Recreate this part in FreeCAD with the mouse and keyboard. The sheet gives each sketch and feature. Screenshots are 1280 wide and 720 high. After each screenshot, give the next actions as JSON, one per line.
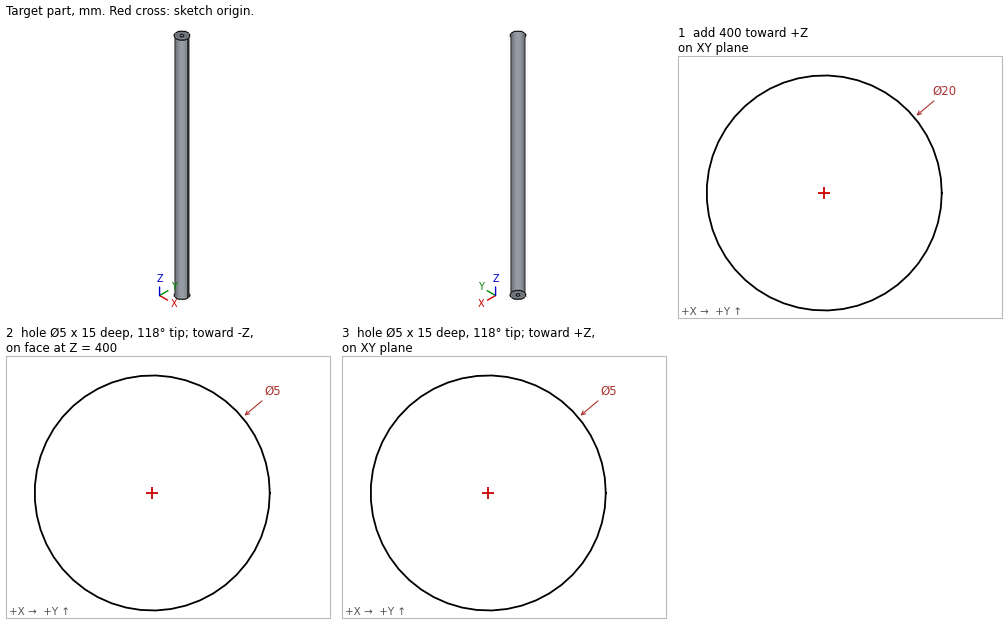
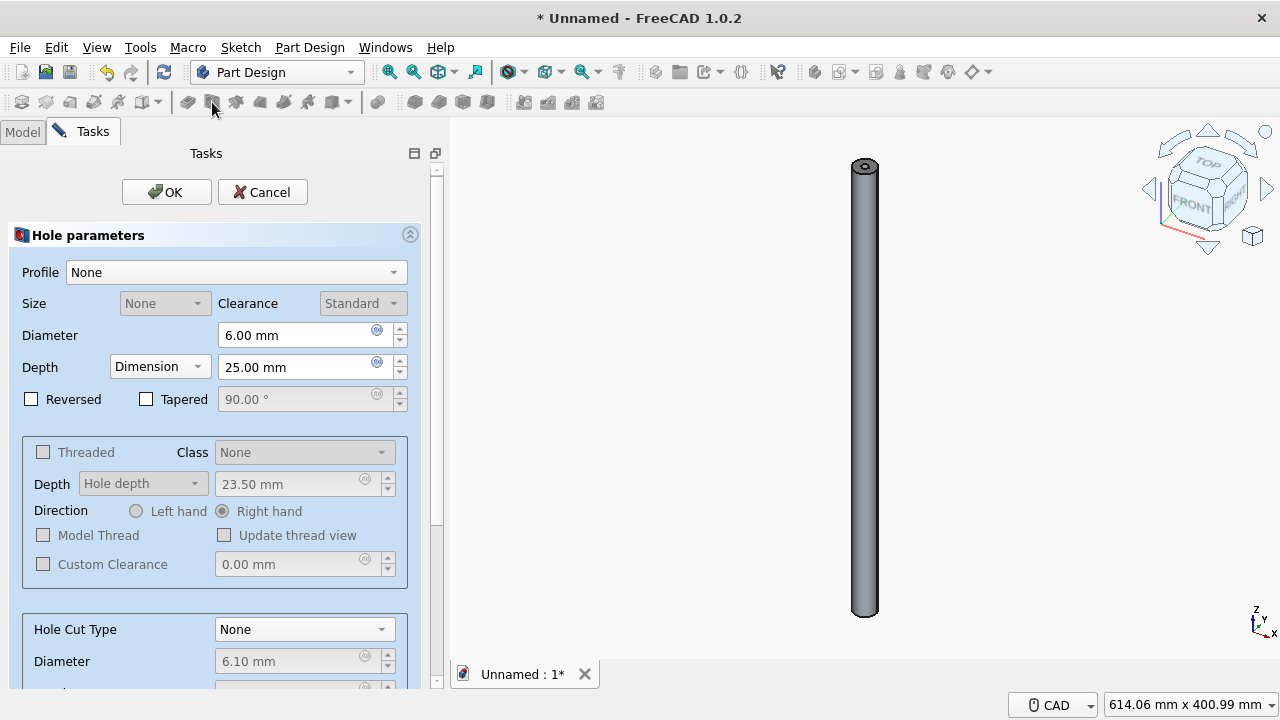
{"action": "triple_click", "coordinate": [305, 335]}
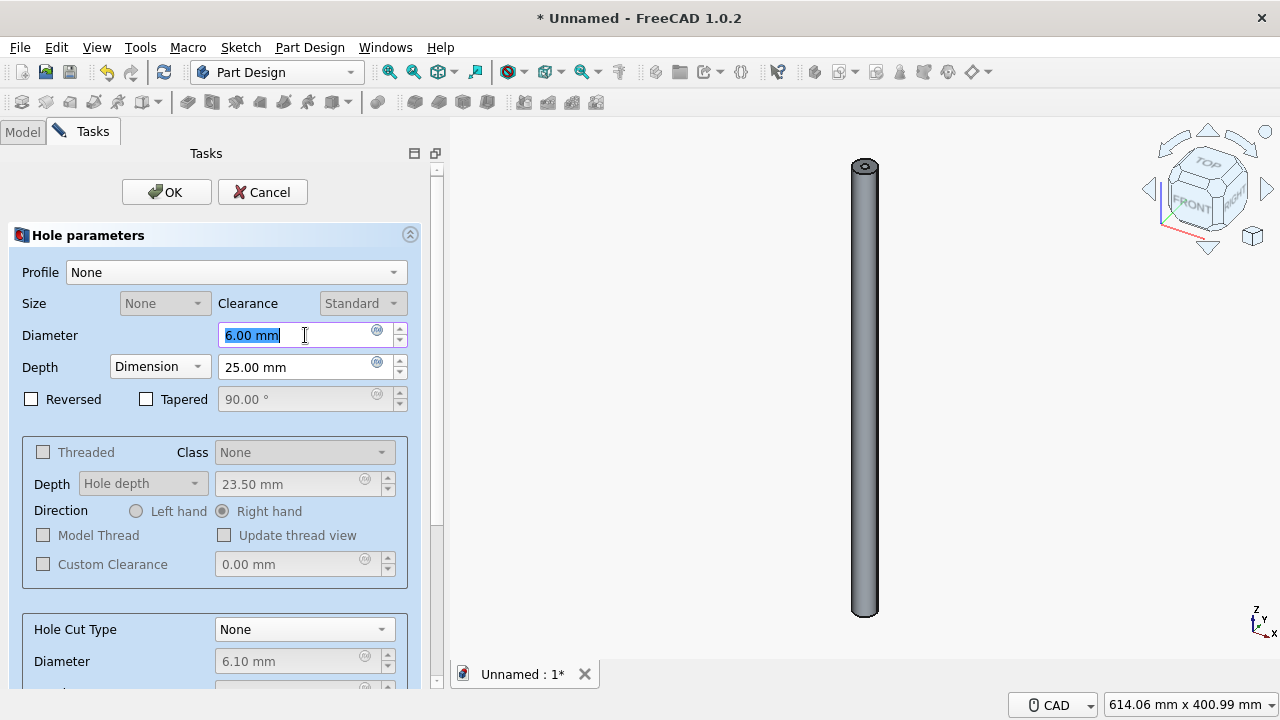
{"action": "type", "text": "5"}
{"action": "key", "text": "Tab"}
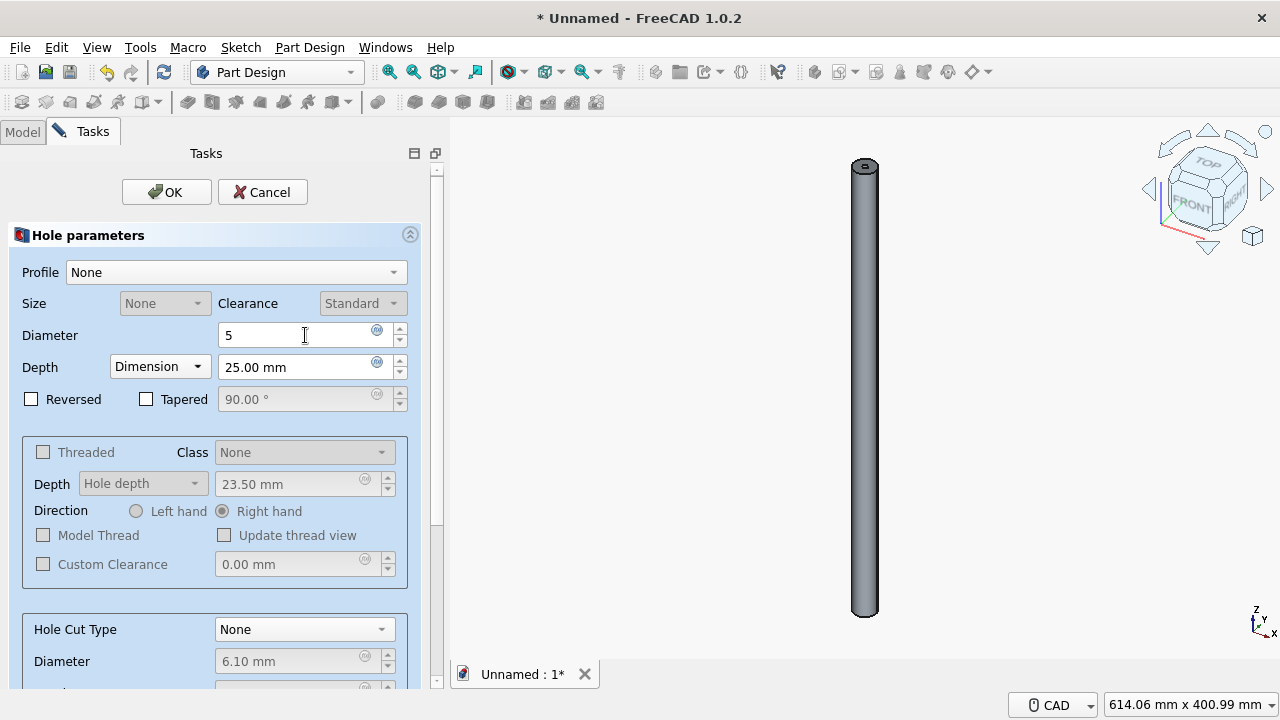
{"action": "triple_click", "coordinate": [305, 367]}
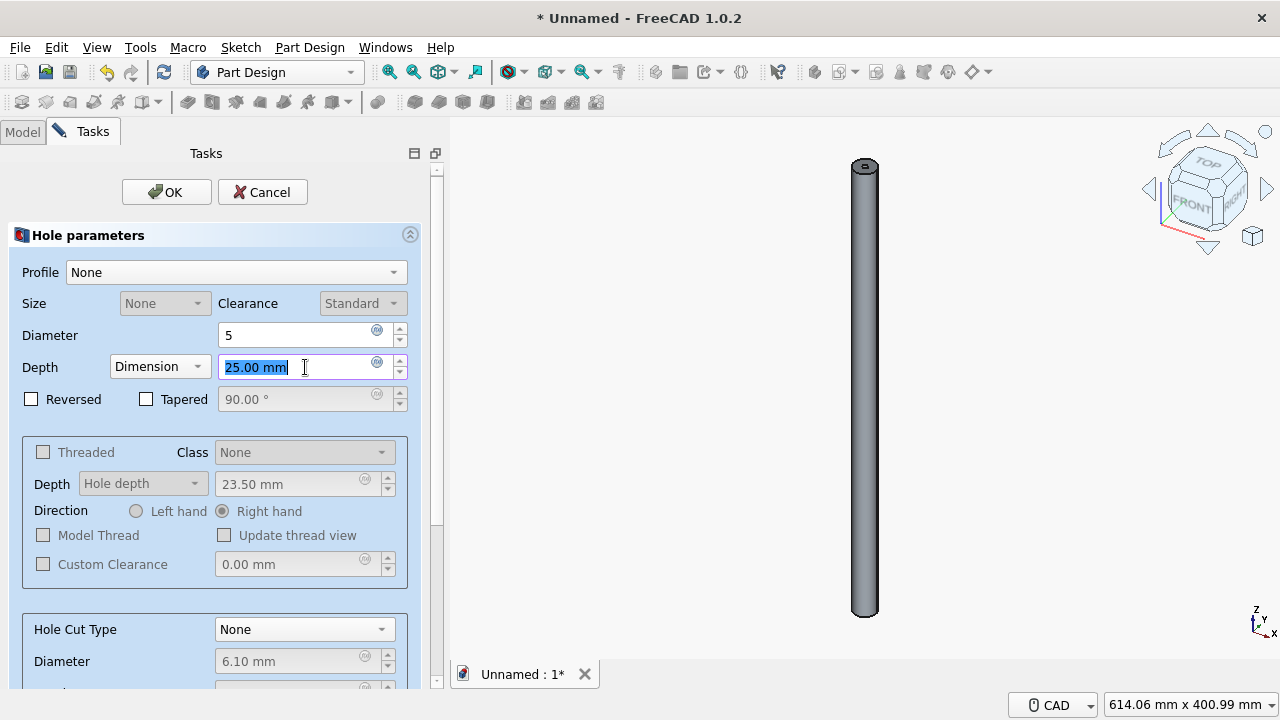
{"action": "type", "text": "15"}
{"action": "key", "text": "Tab"}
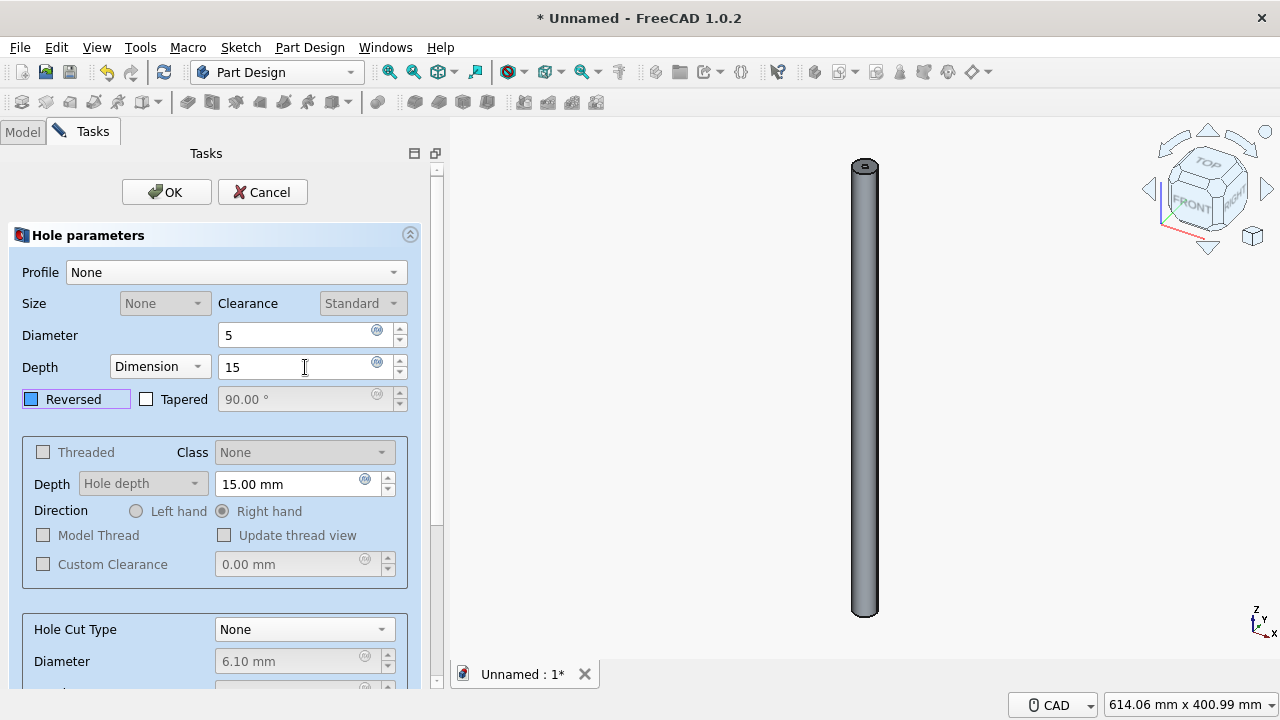
{"action": "left_click", "coordinate": [167, 192]}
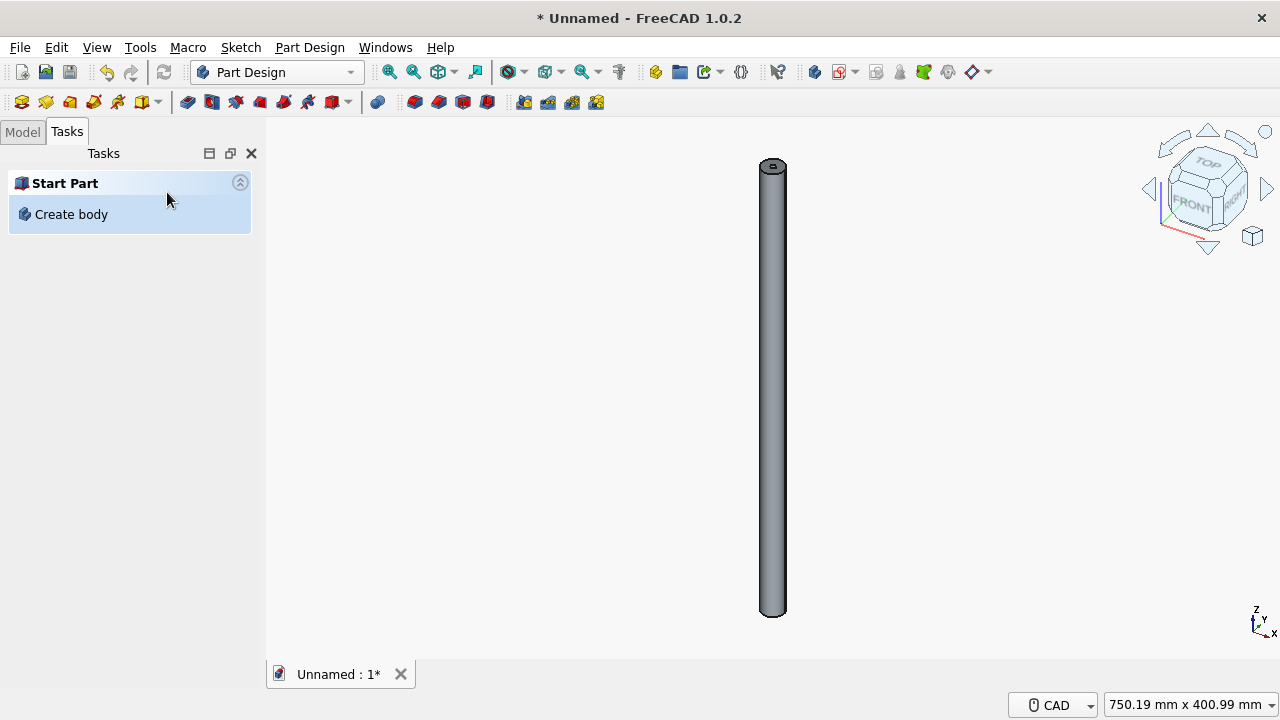
{"action": "left_click", "coordinate": [840, 72]}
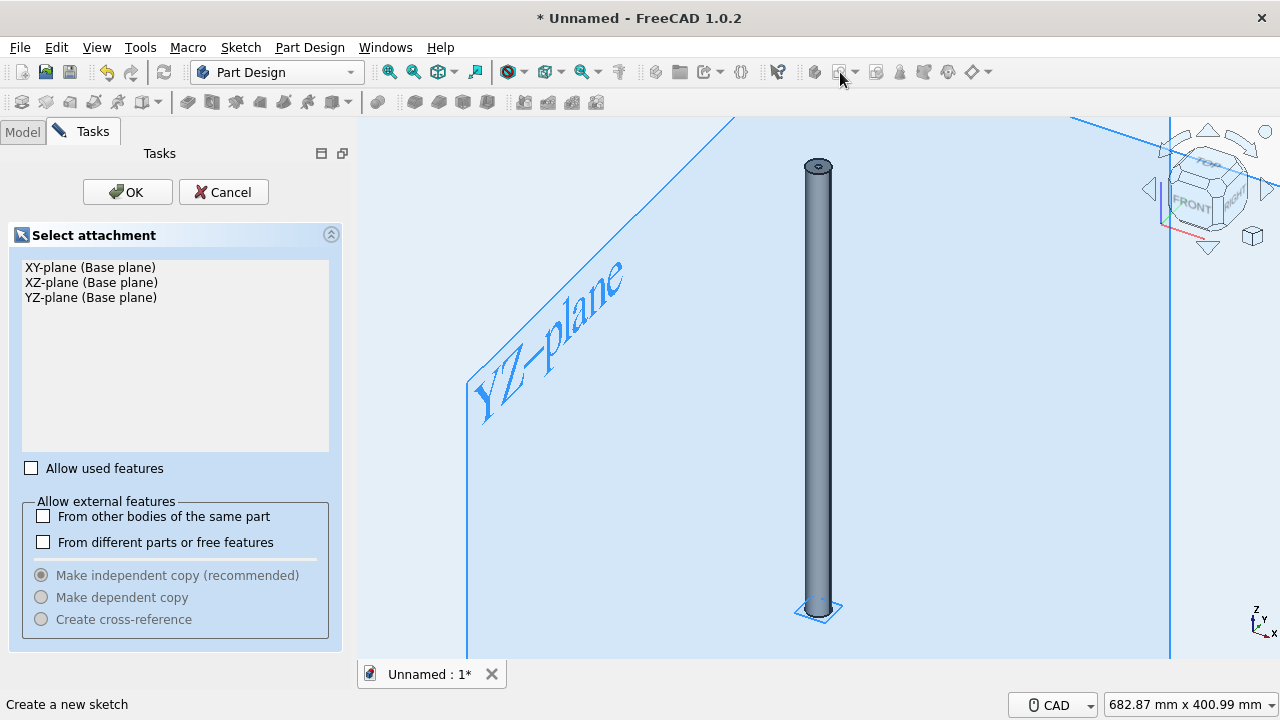
{"action": "left_click", "coordinate": [82, 268]}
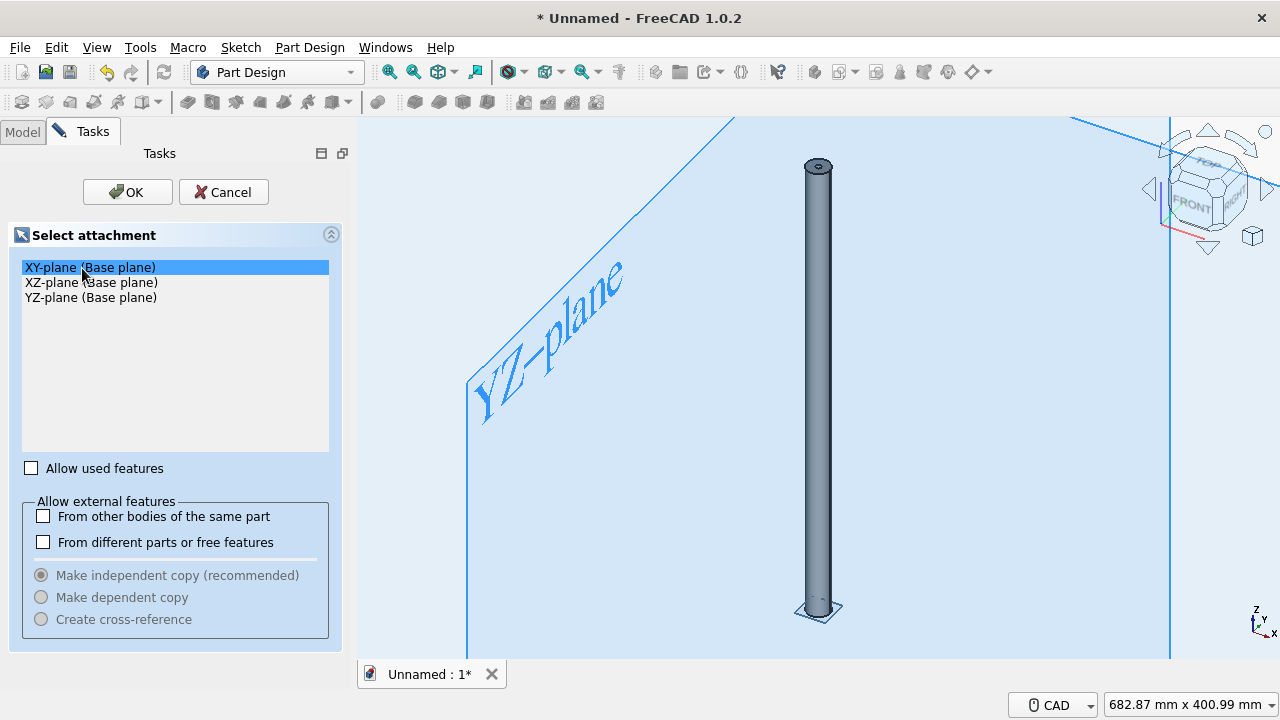
{"action": "left_click", "coordinate": [128, 192]}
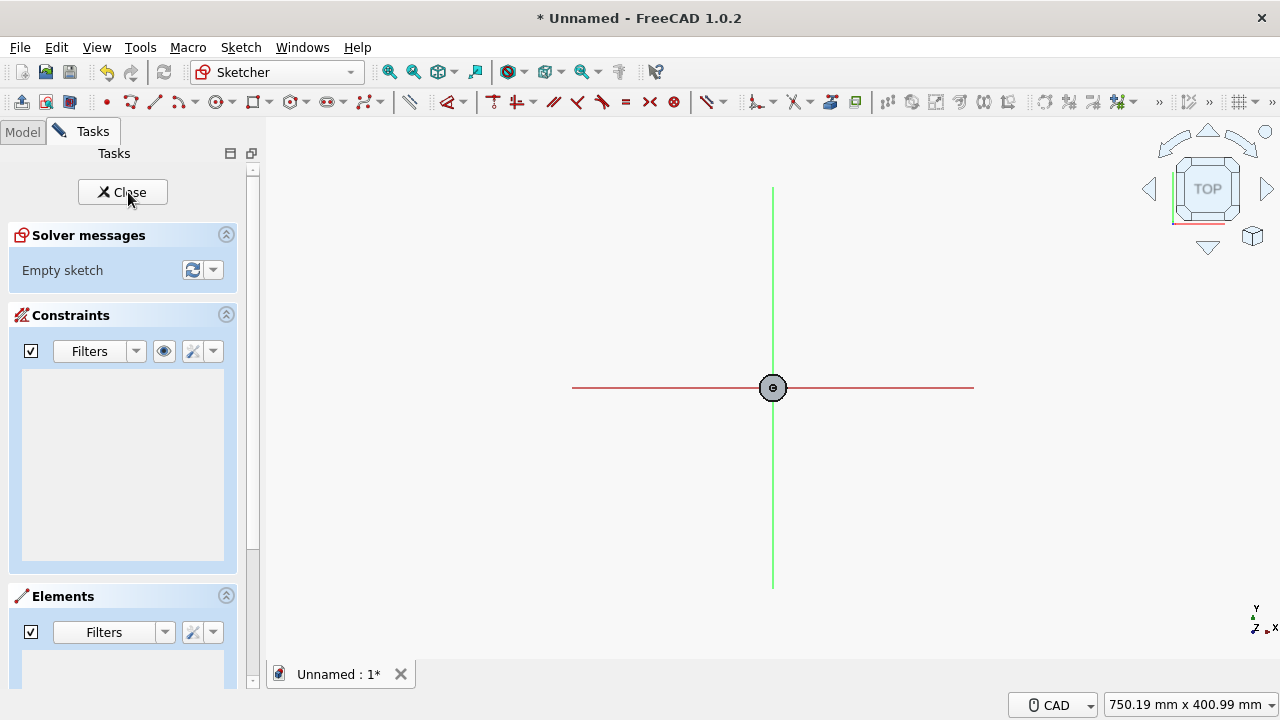
{"action": "left_click", "coordinate": [70, 102]}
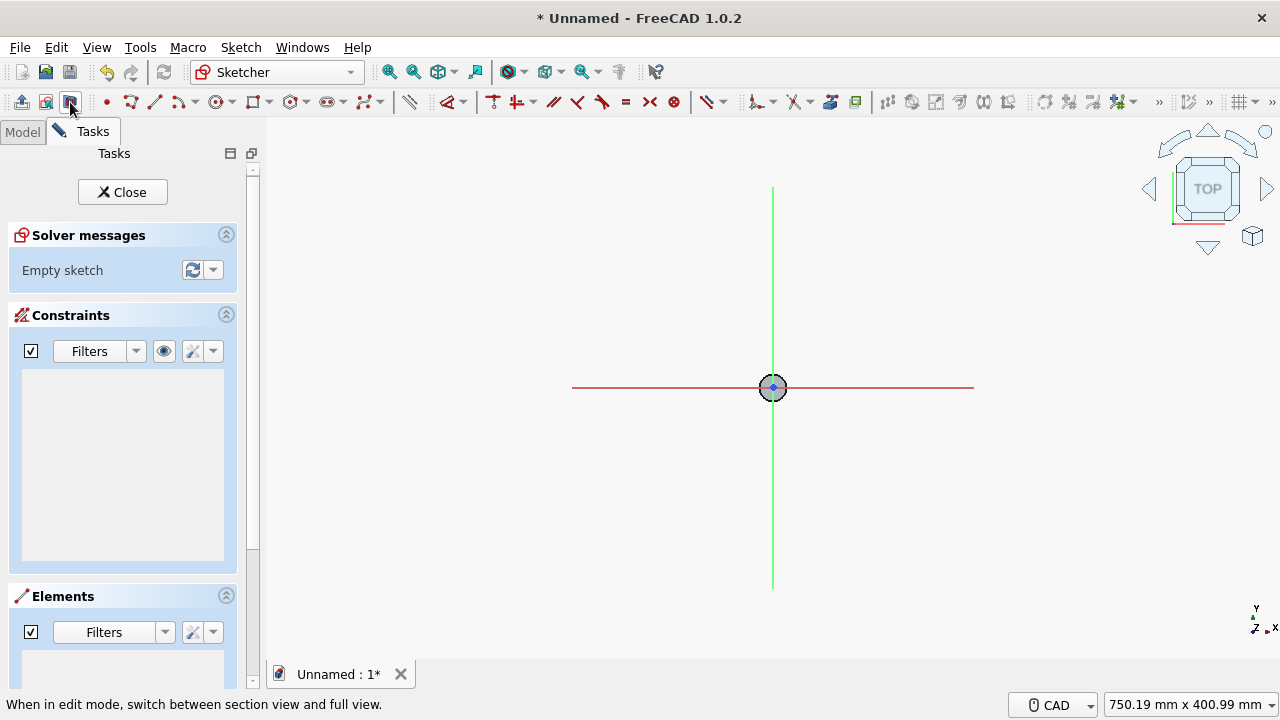
{"action": "scroll", "coordinate": [777, 388], "scroll_direction": "up", "scroll_amount": 15}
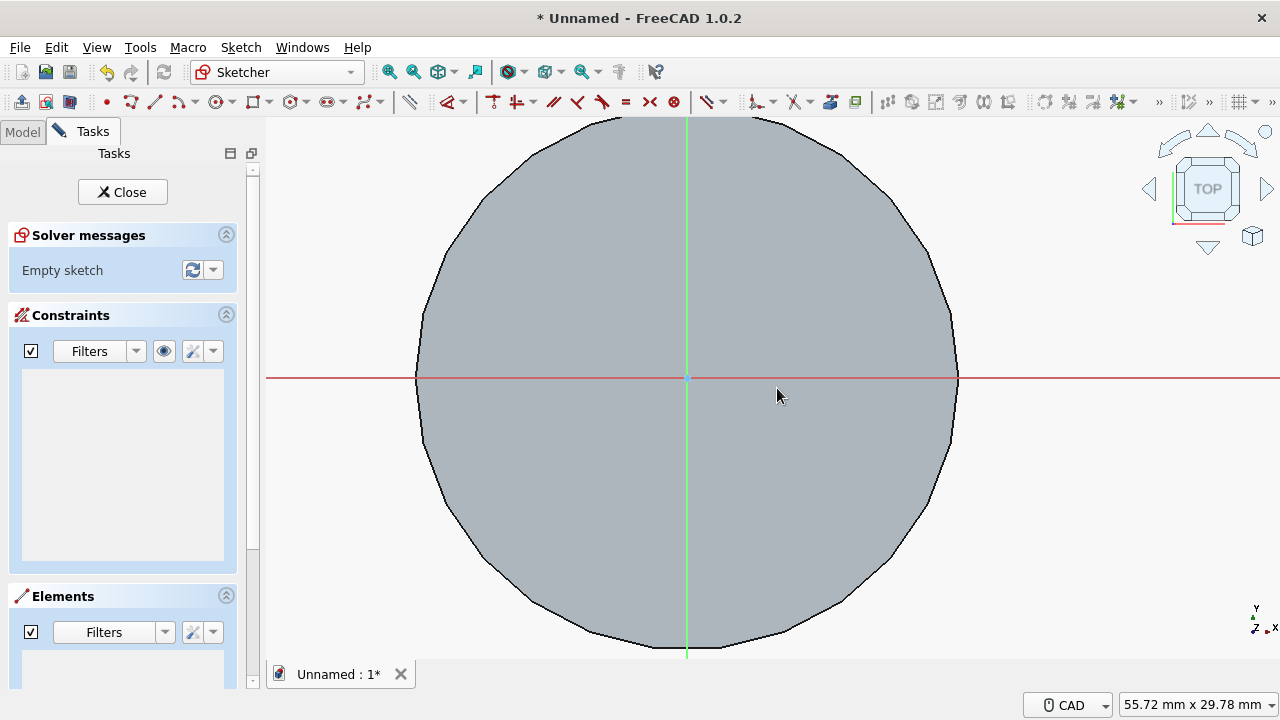
{"action": "scroll", "coordinate": [677, 373], "scroll_direction": "up", "scroll_amount": 5}